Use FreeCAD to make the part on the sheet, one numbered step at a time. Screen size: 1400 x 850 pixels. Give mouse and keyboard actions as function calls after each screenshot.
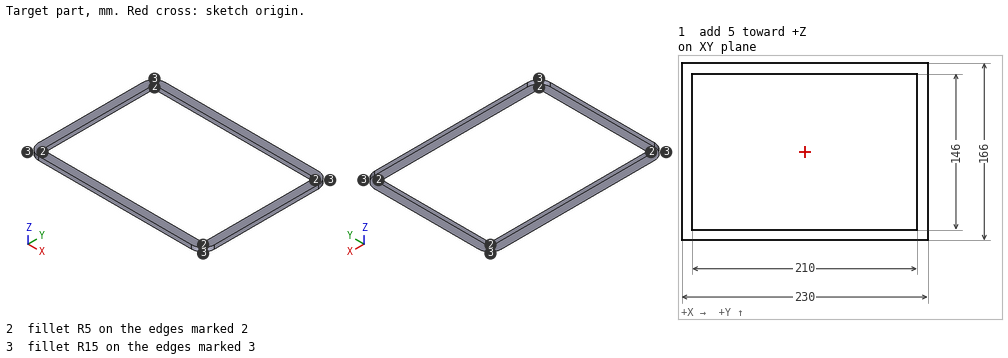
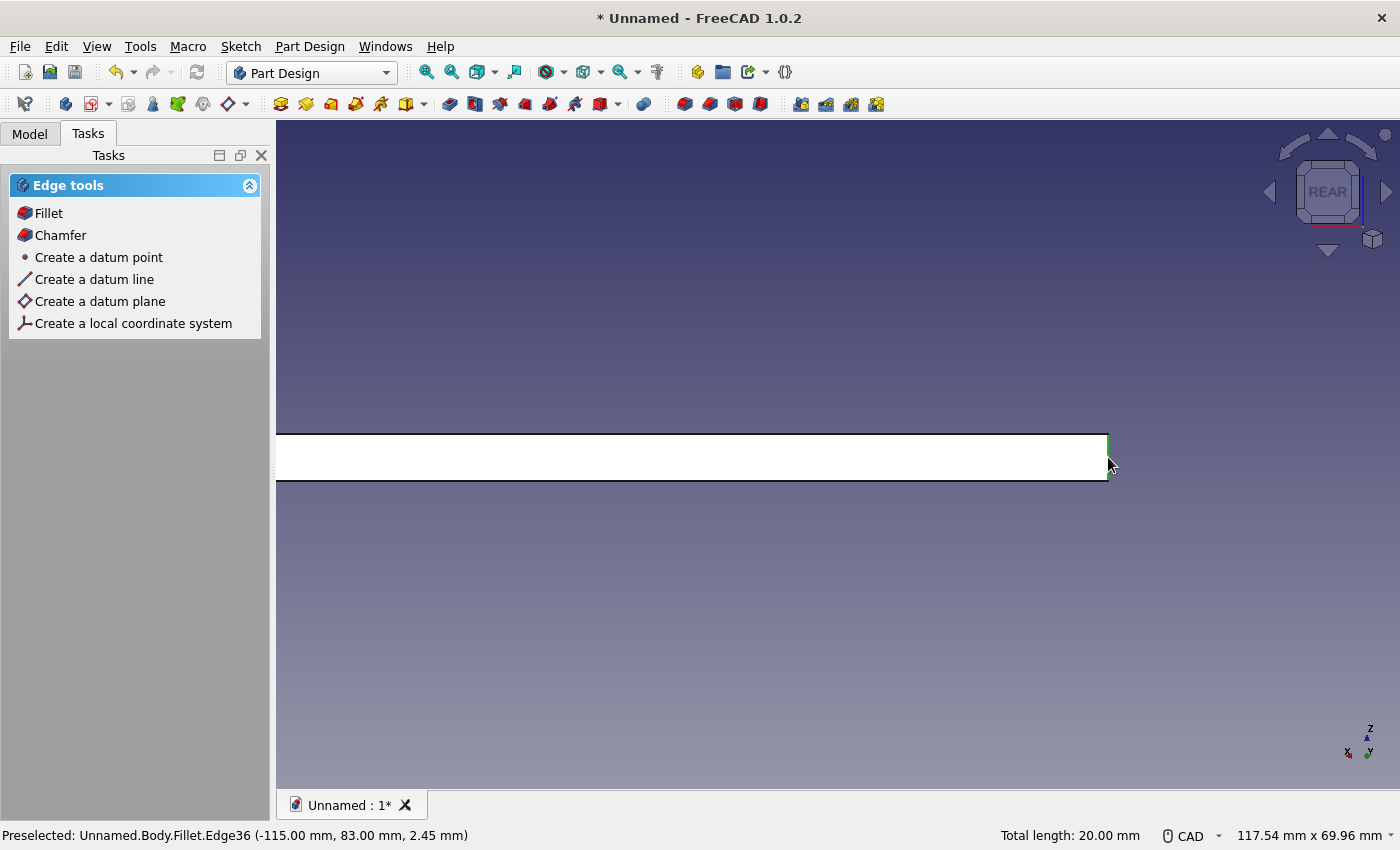
click(685, 104)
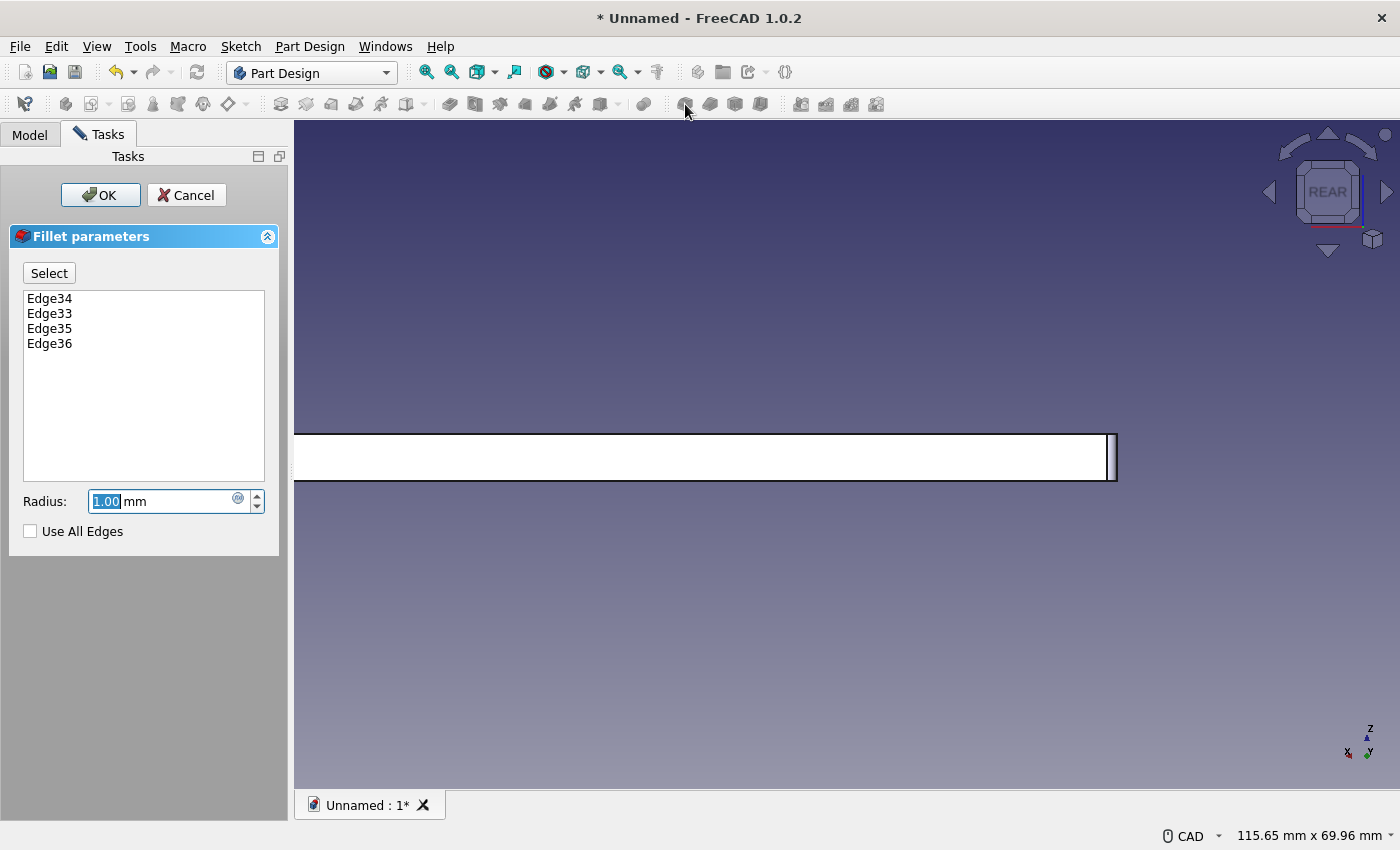
text(15)
key(Tab)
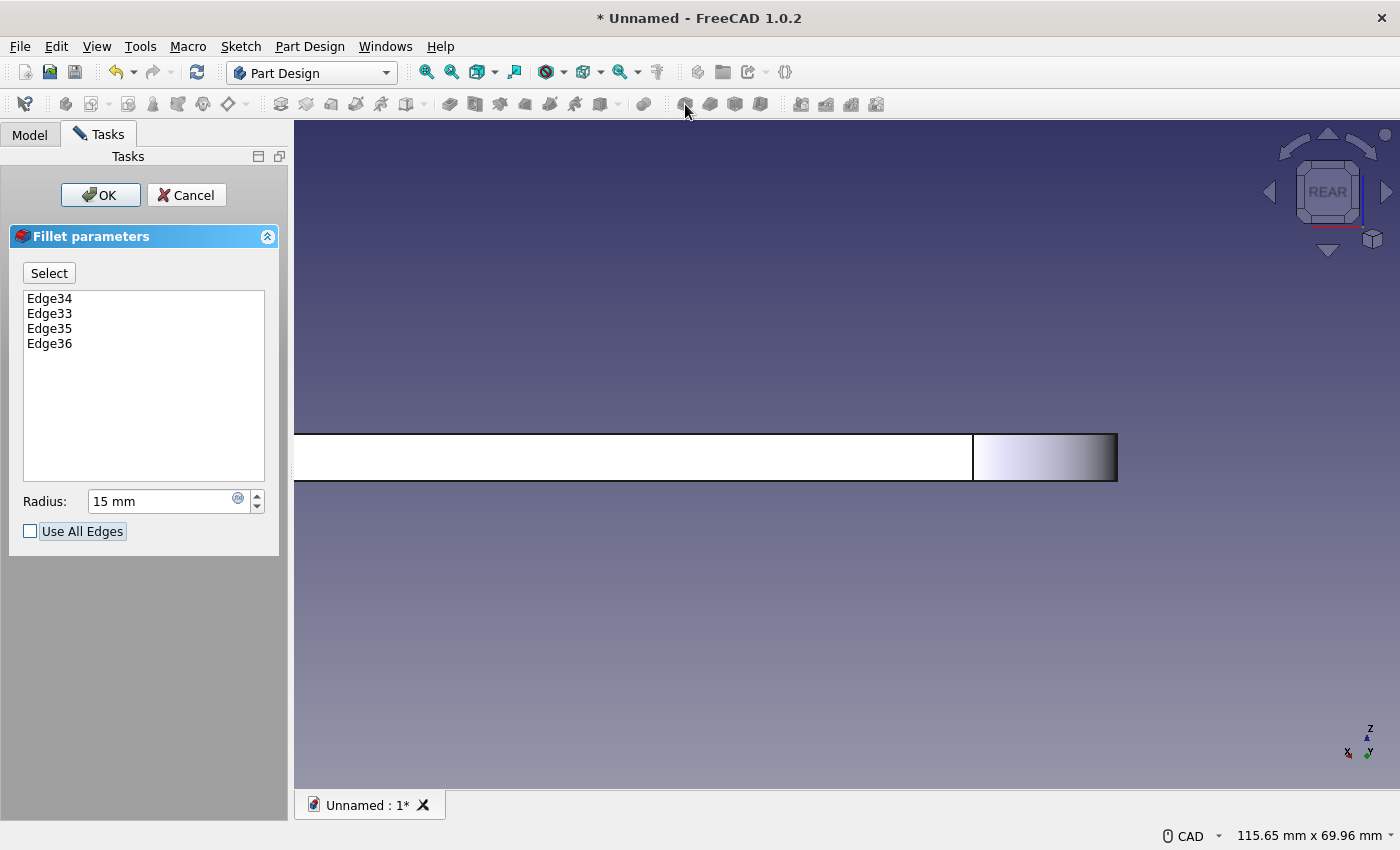
click(101, 195)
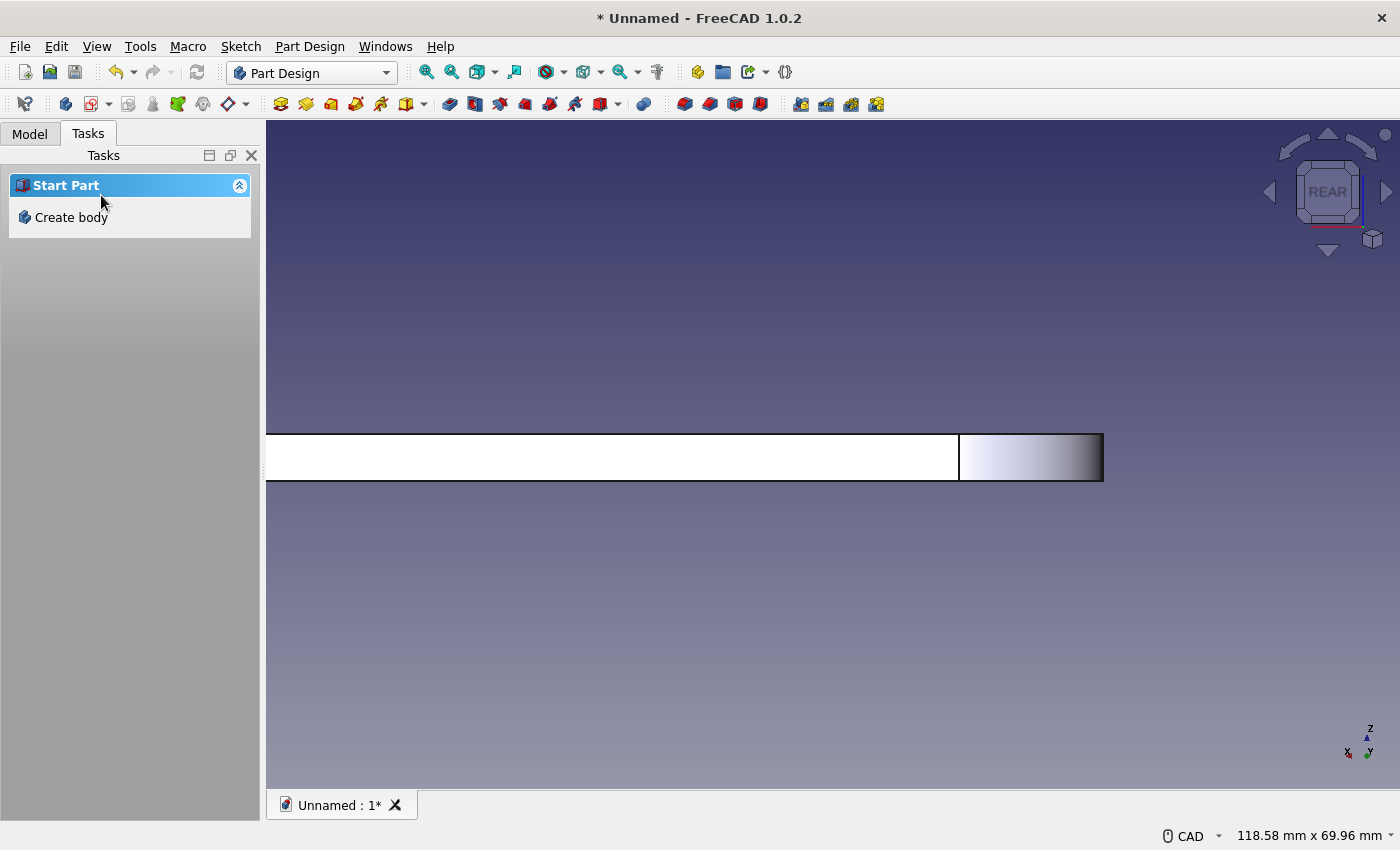
key(0)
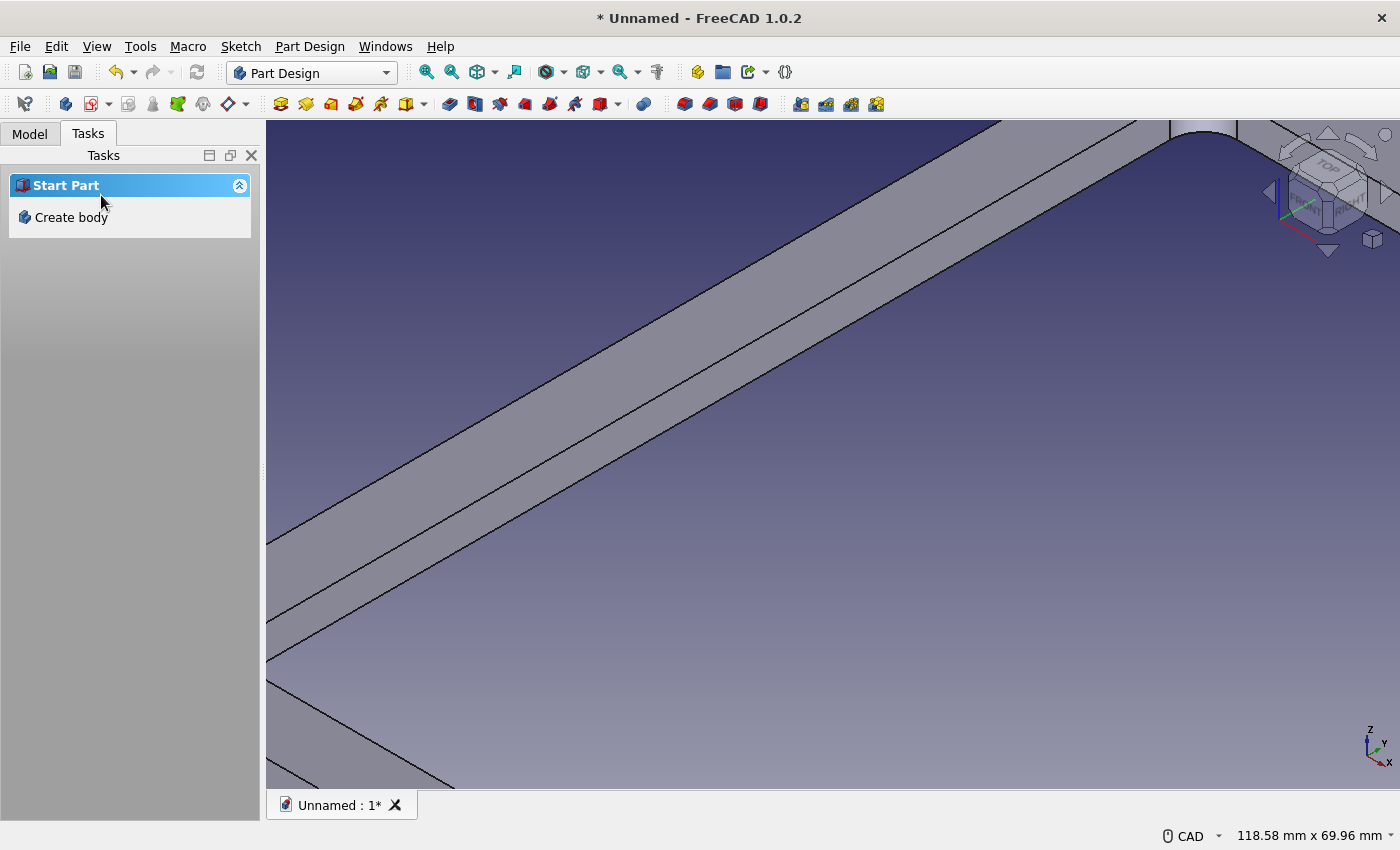
key(v)
key(f)